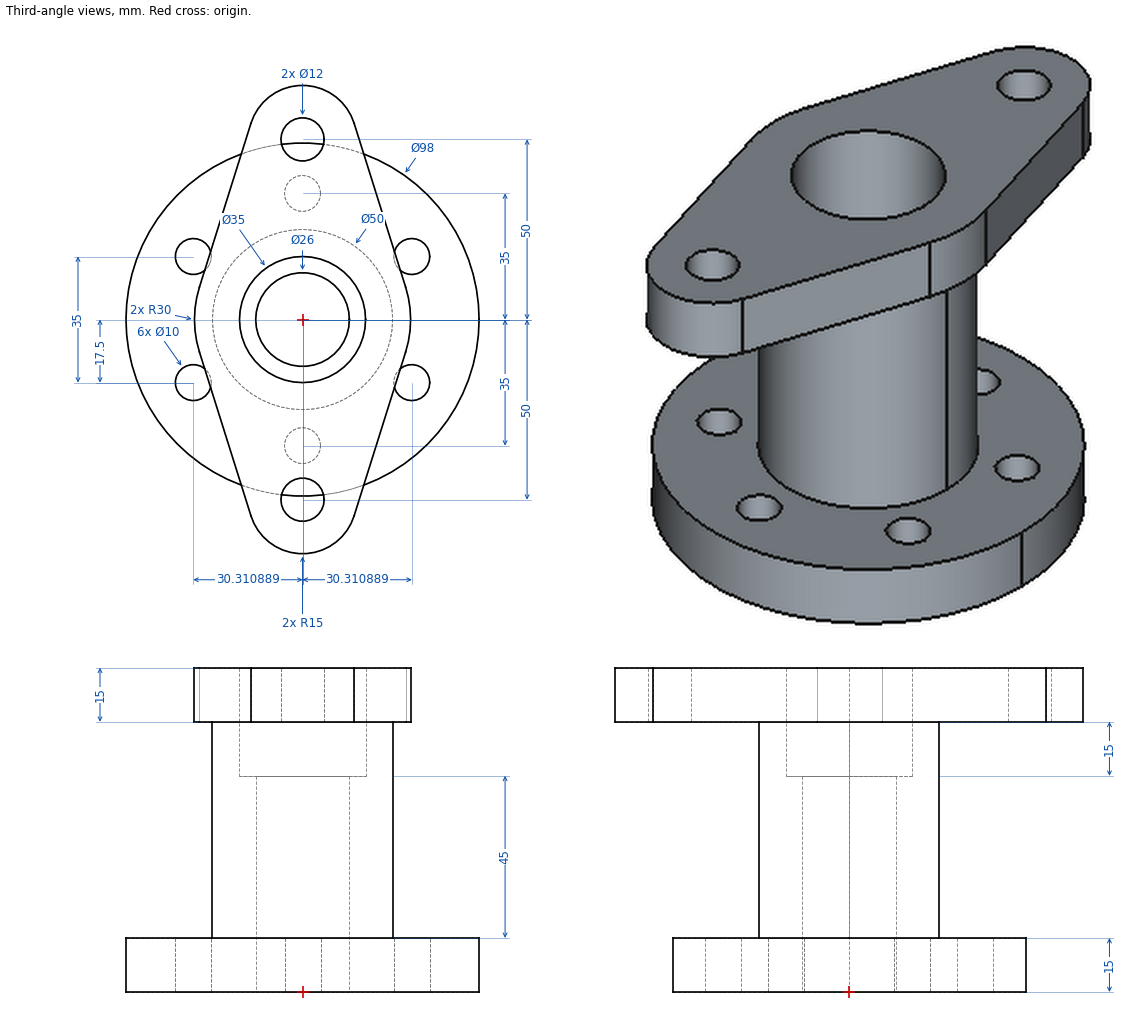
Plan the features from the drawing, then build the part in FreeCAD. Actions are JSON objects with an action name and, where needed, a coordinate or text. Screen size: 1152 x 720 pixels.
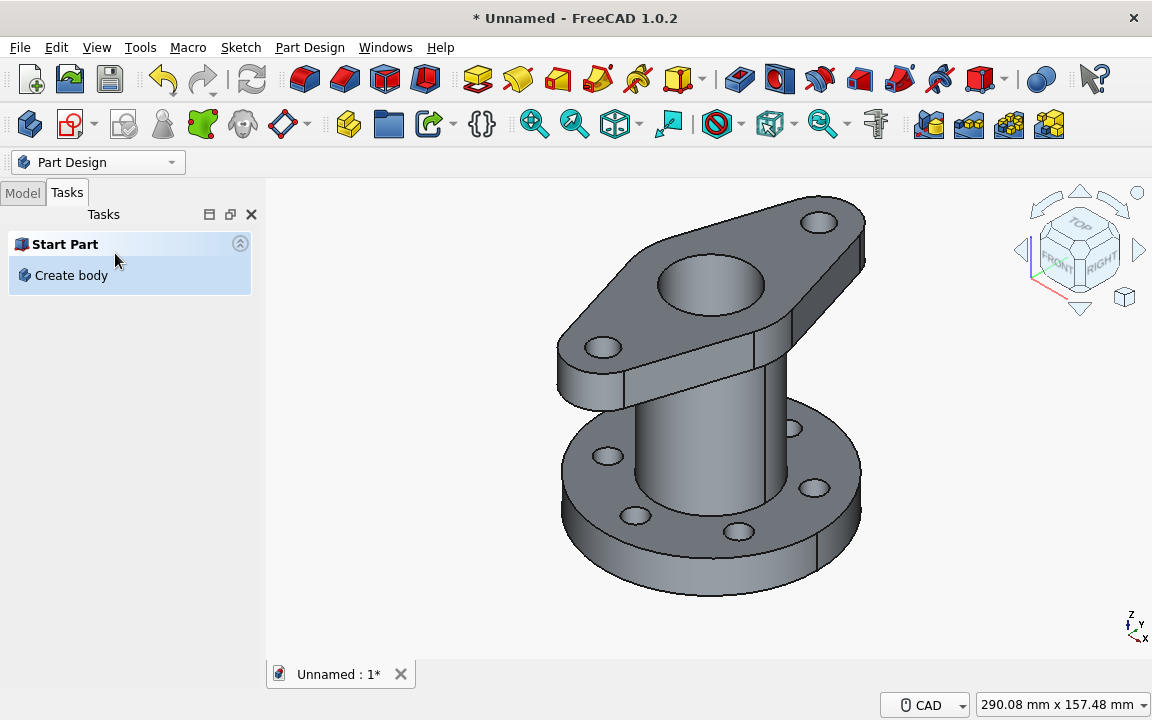
{"action": "left_click", "coordinate": [536, 124]}